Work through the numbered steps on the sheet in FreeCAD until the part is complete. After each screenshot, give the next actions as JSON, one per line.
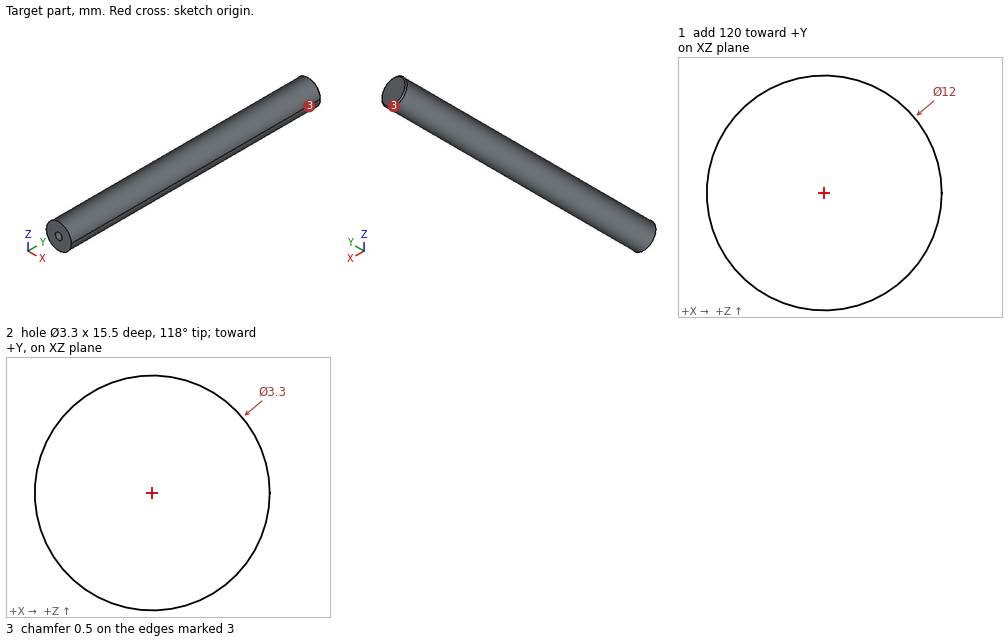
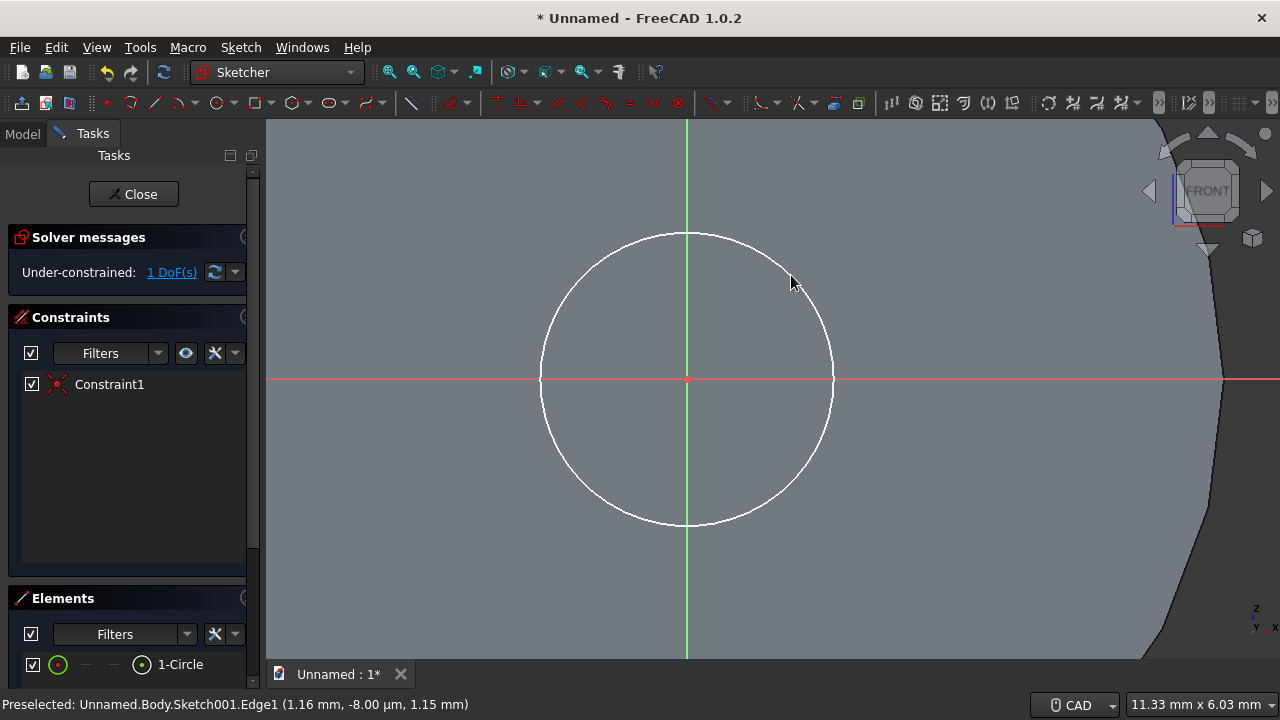
{"action": "left_click", "coordinate": [450, 104]}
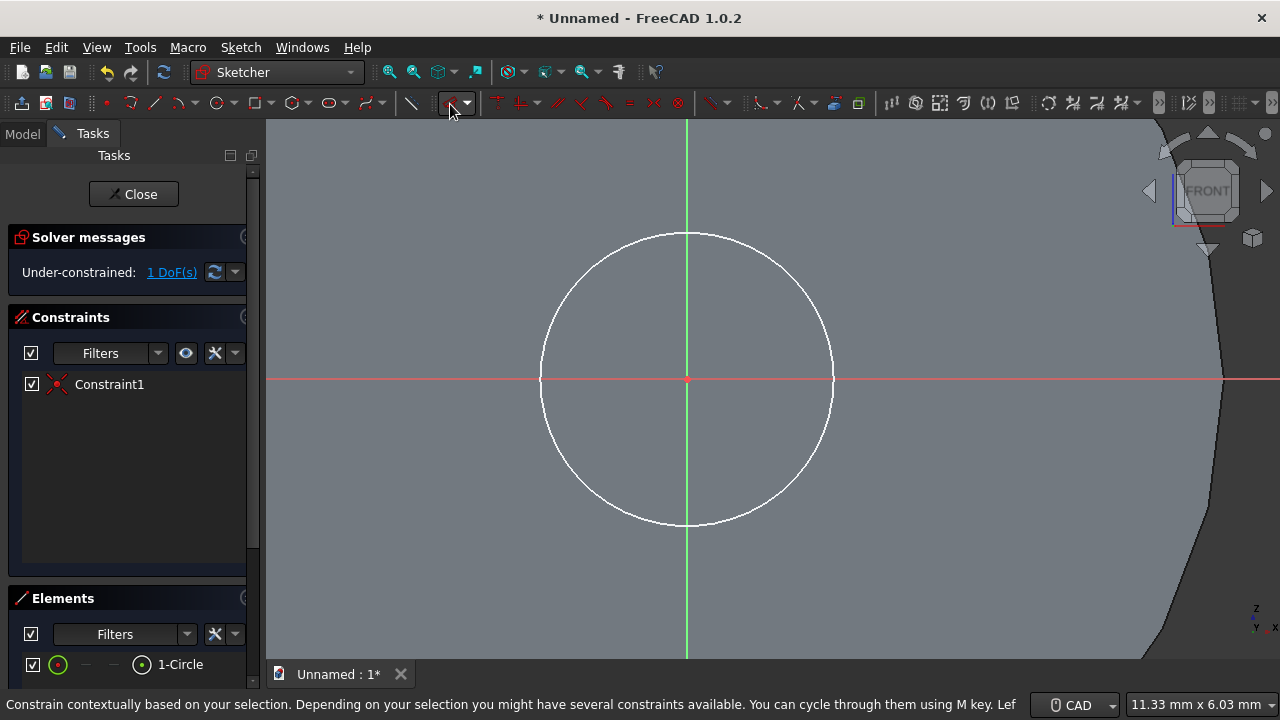
{"action": "left_click", "coordinate": [790, 275]}
{"action": "left_click", "coordinate": [812, 252]}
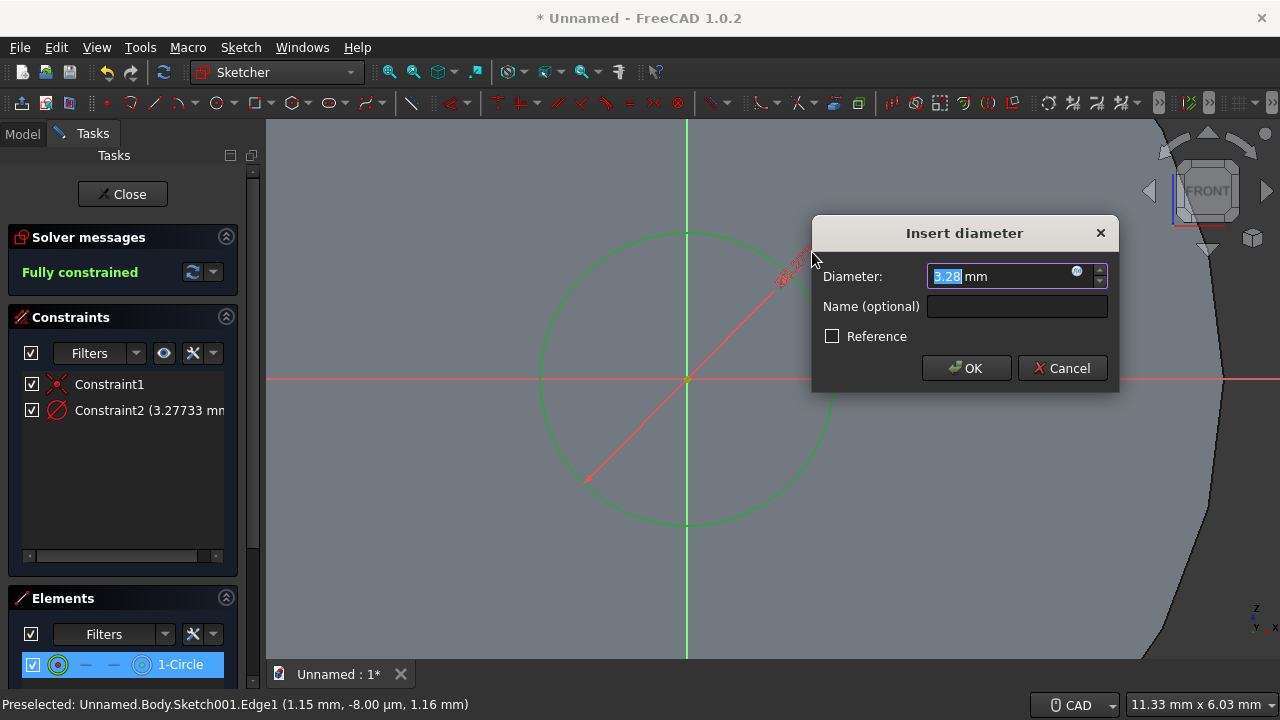
{"action": "type", "text": "3.3"}
{"action": "key", "text": "Return"}
{"action": "key", "text": "Escape"}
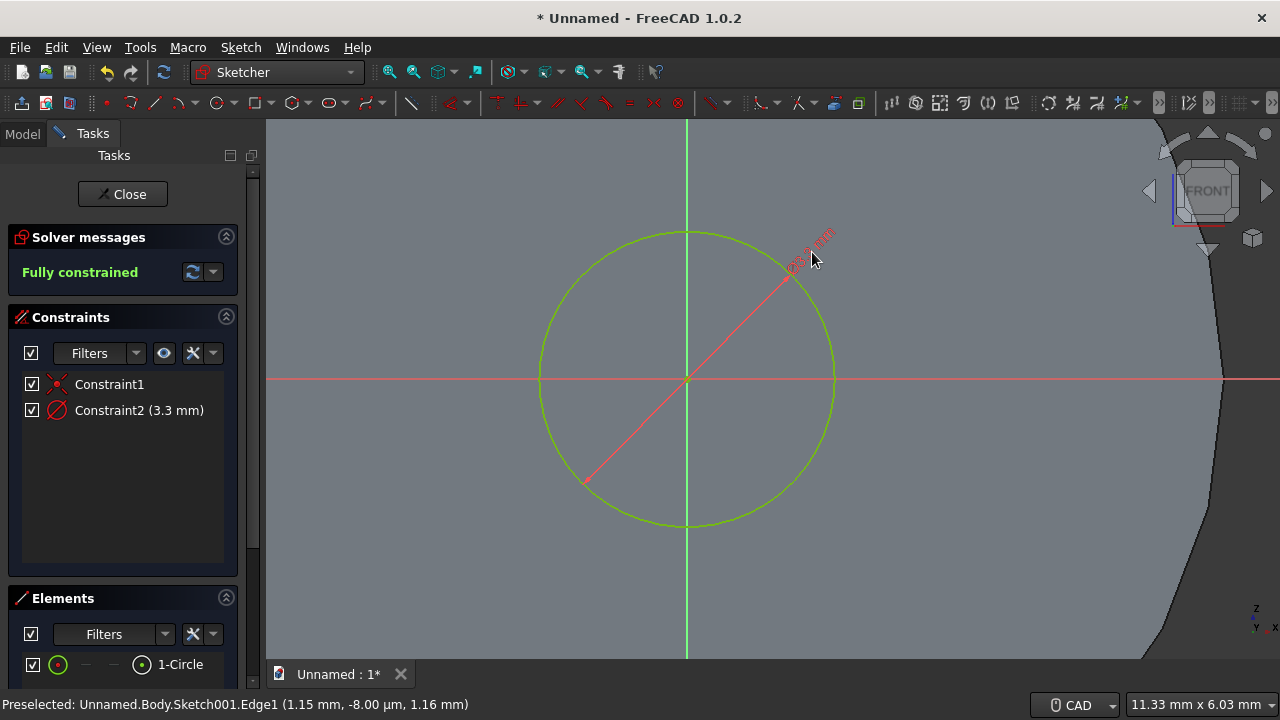
{"action": "left_click", "coordinate": [123, 194]}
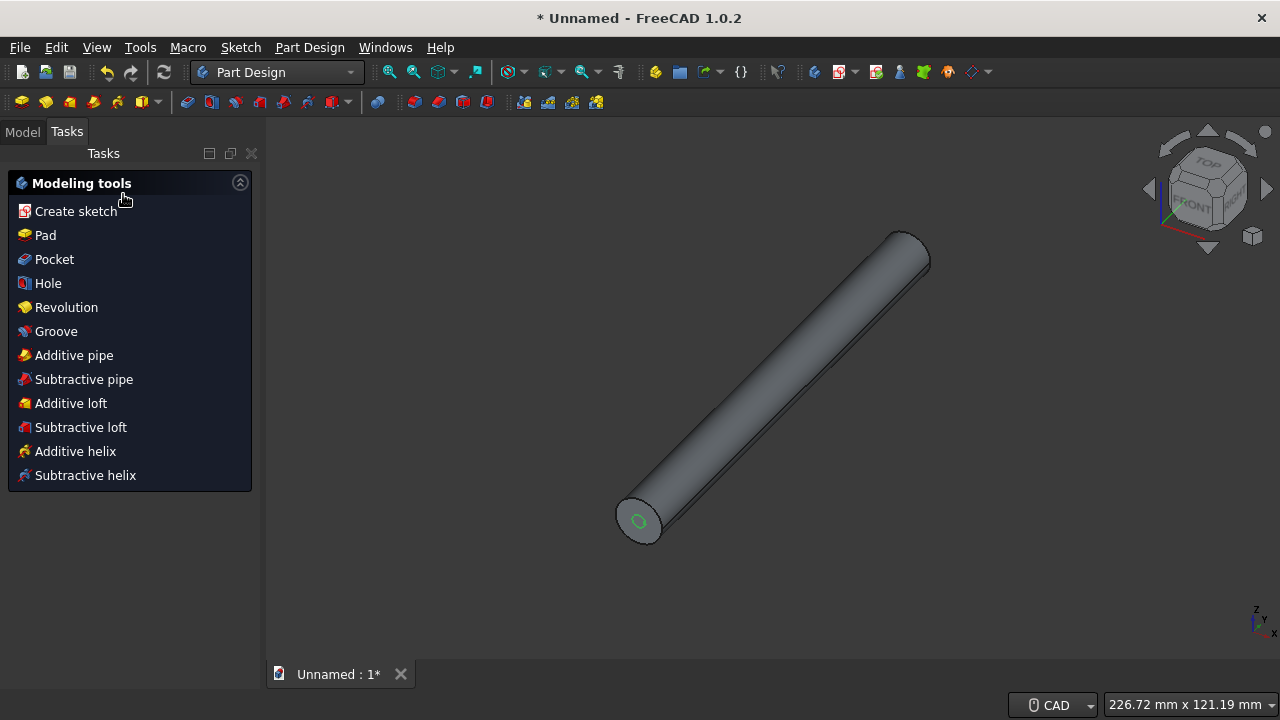
{"action": "left_click", "coordinate": [212, 102]}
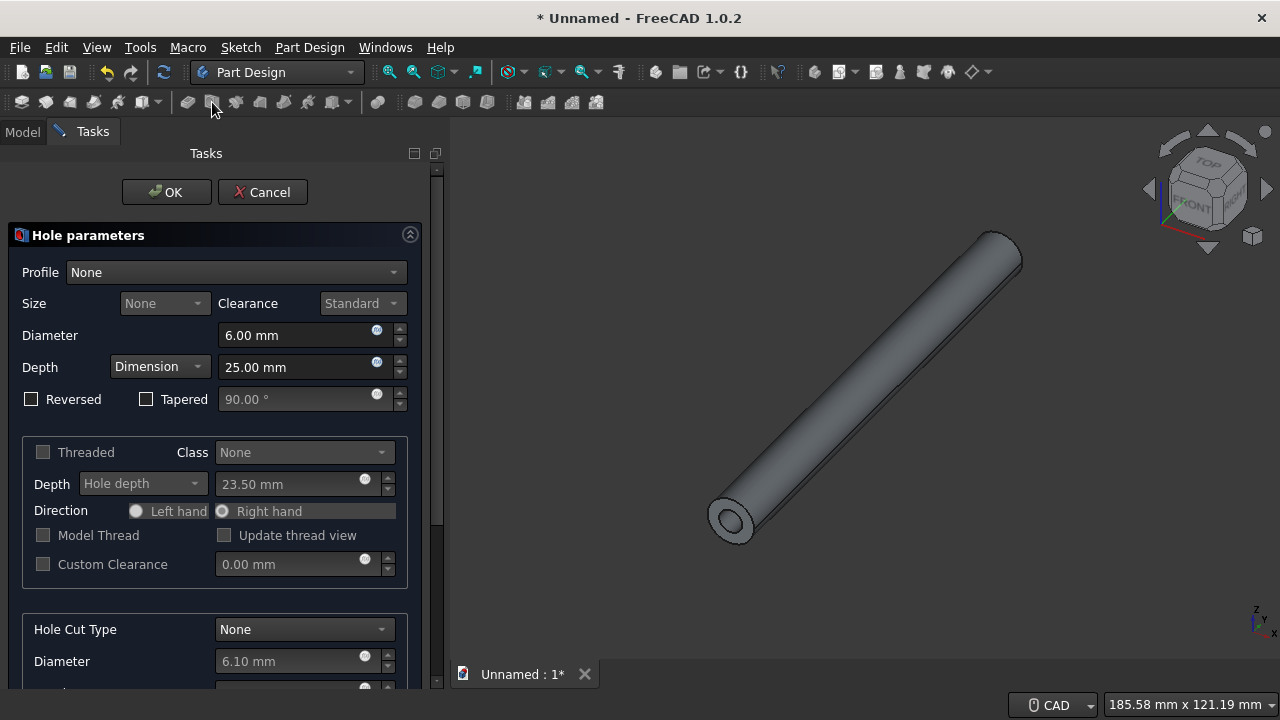
{"action": "triple_click", "coordinate": [305, 335]}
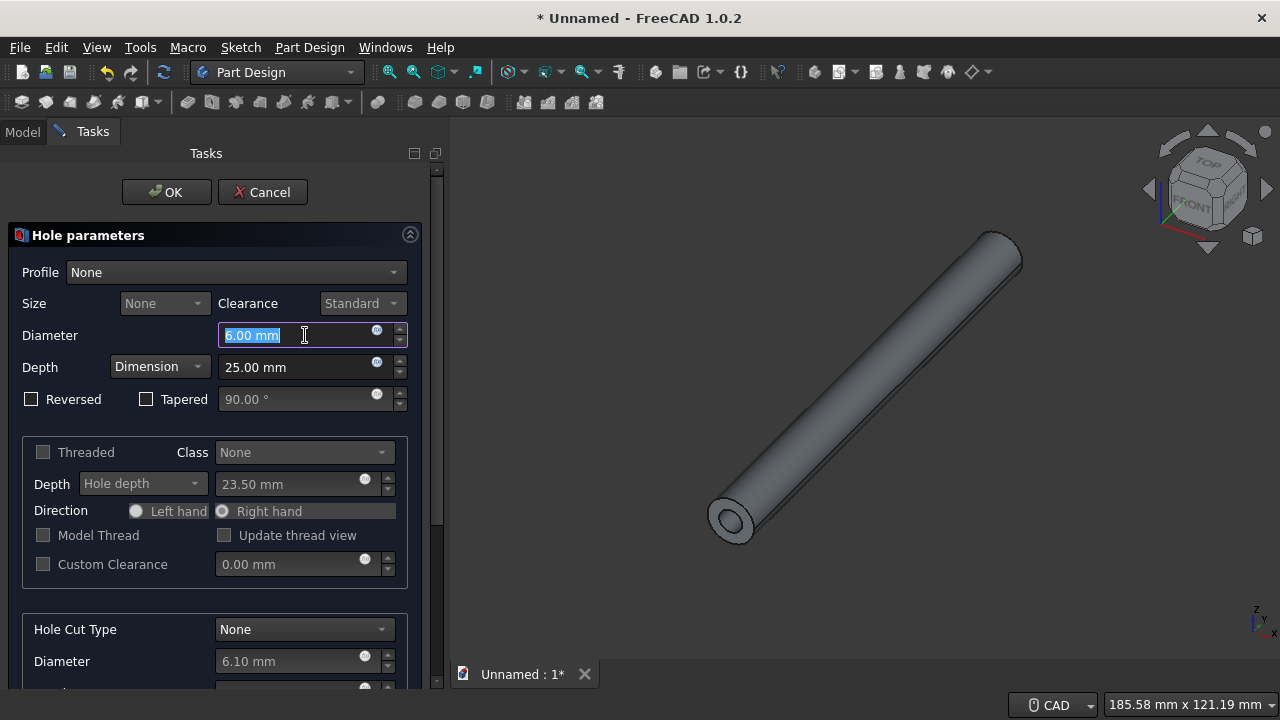
{"action": "type", "text": "3.3"}
{"action": "key", "text": "Tab"}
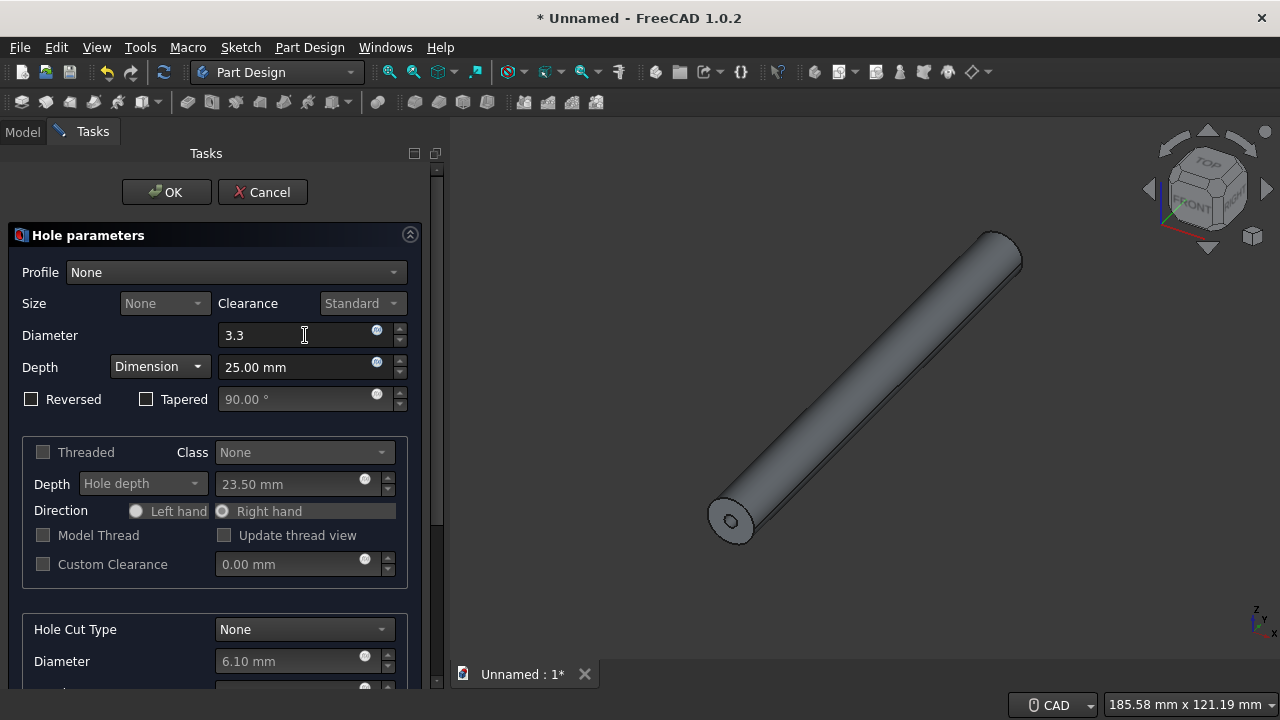
{"action": "triple_click", "coordinate": [305, 367]}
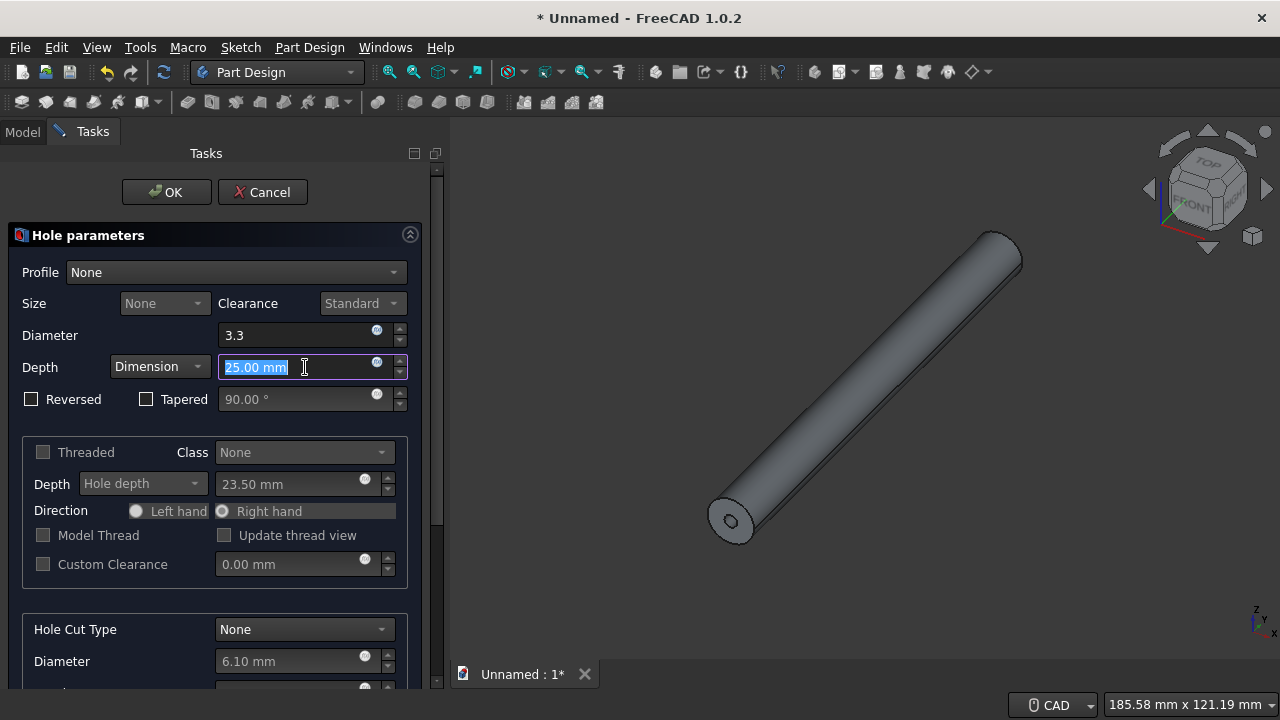
{"action": "type", "text": "15.5"}
{"action": "key", "text": "Tab"}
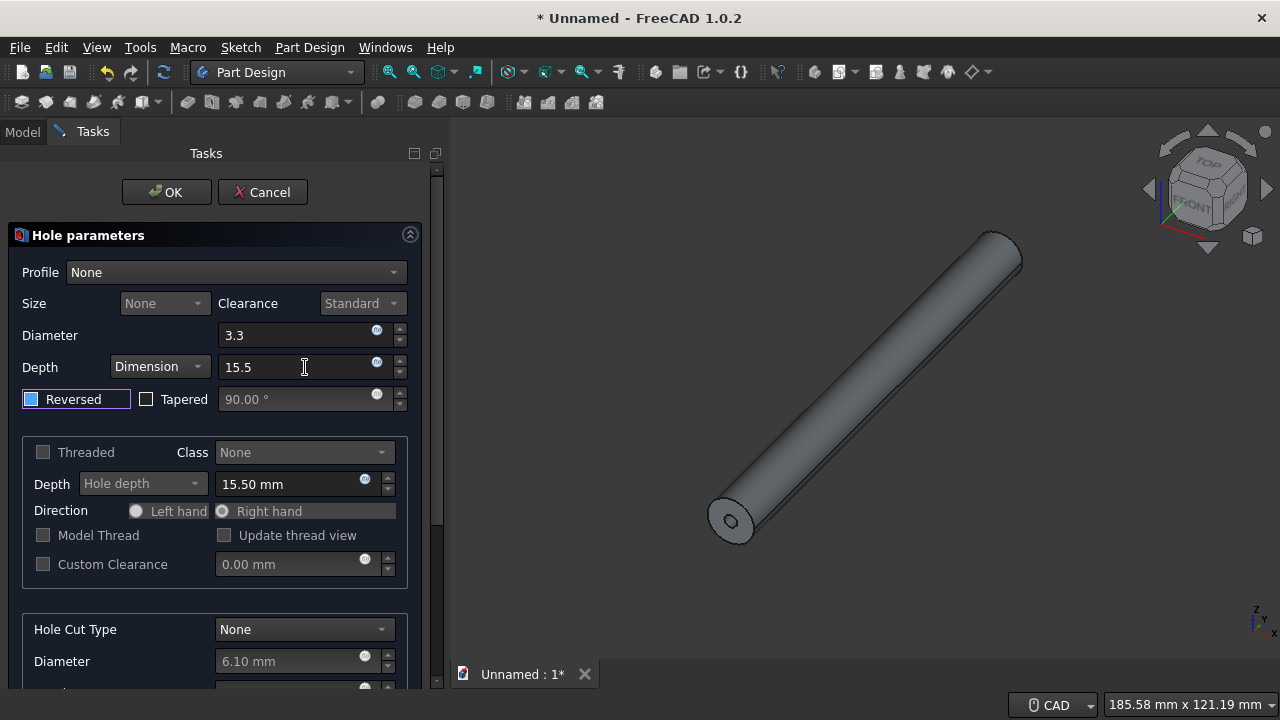
{"action": "left_click", "coordinate": [167, 192]}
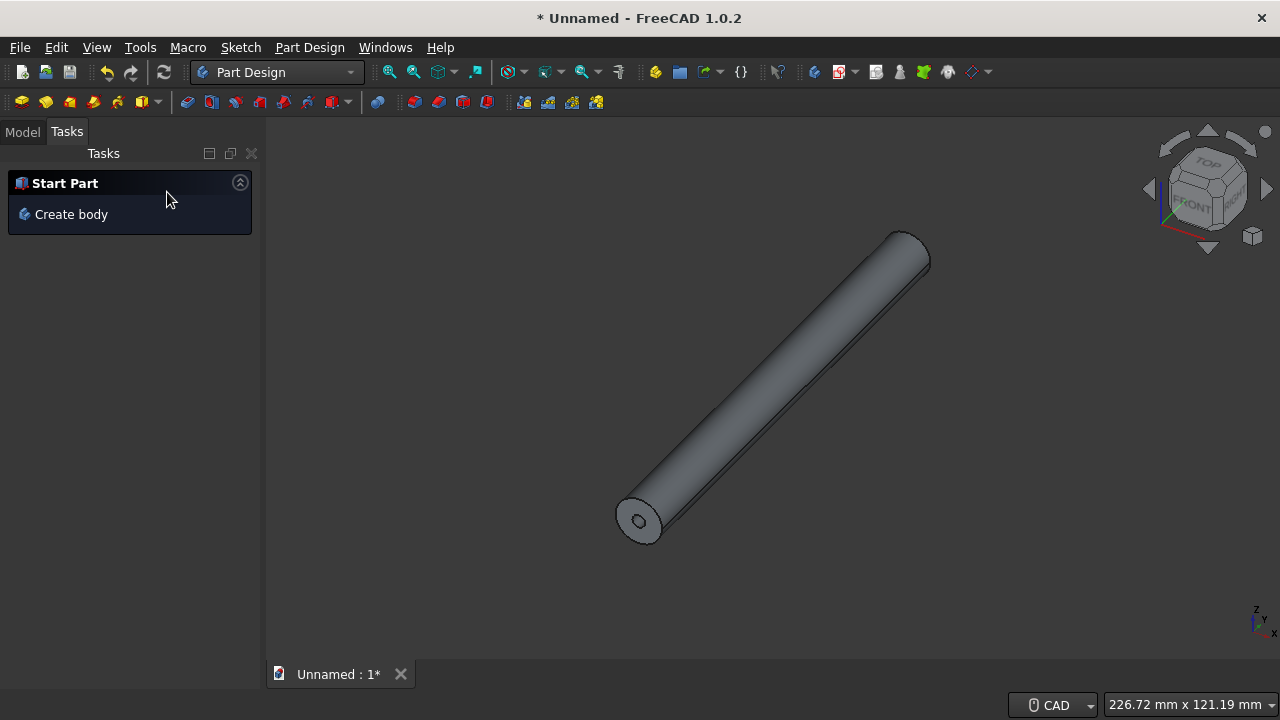
{"action": "key", "text": "0"}